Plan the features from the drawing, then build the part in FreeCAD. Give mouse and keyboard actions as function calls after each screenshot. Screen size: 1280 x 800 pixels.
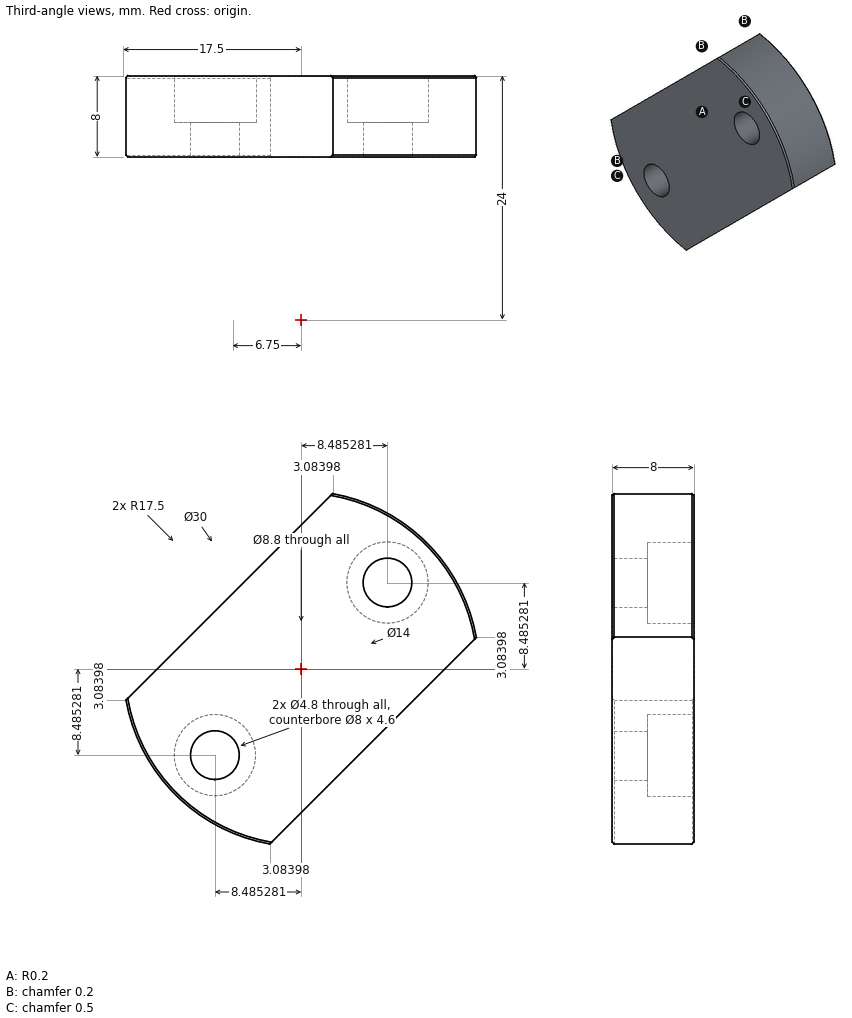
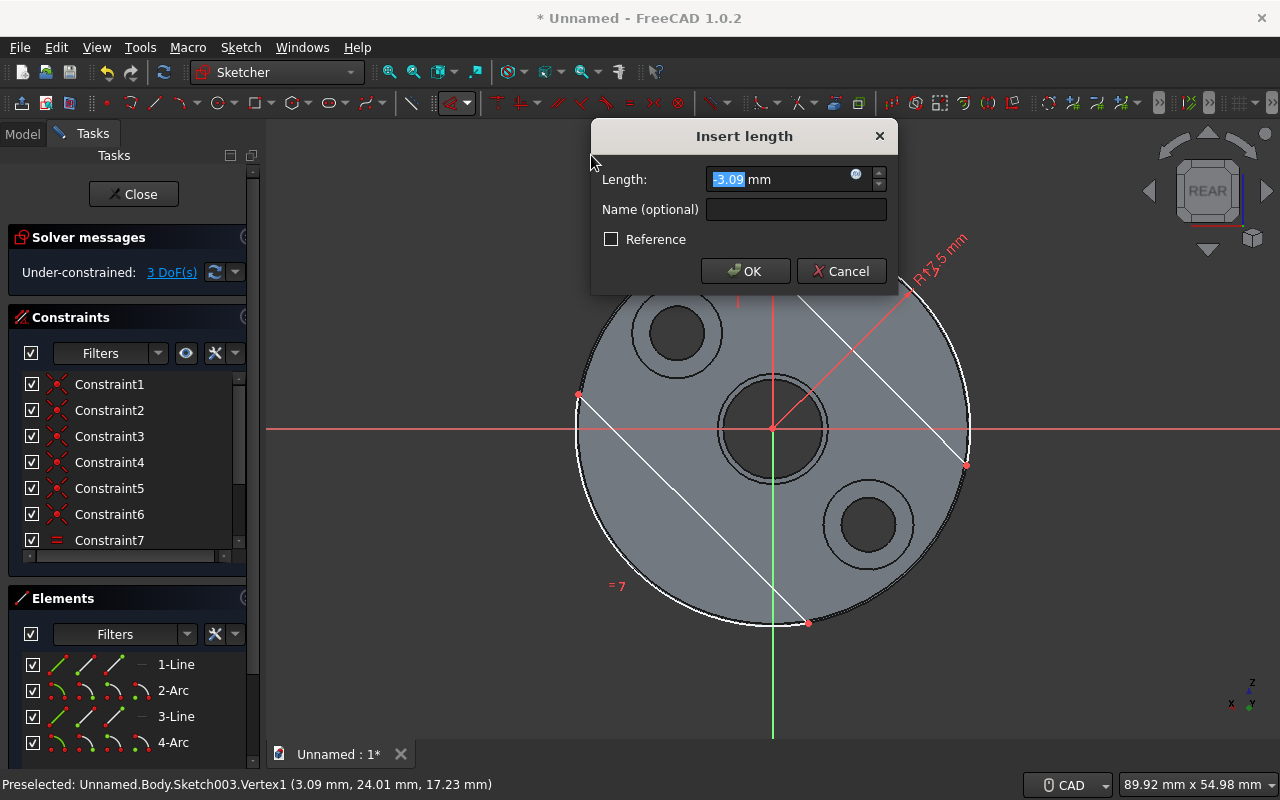
text(-3.08398)
key(Return)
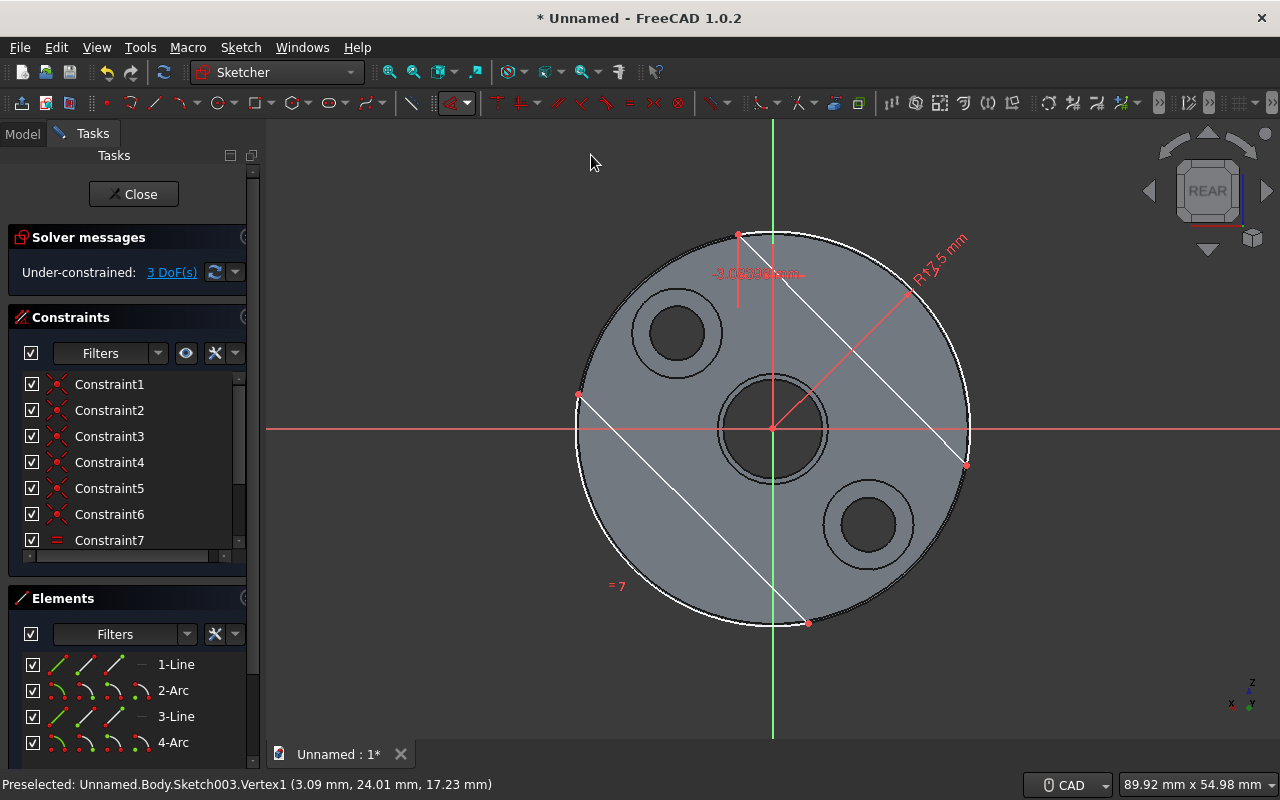
click(967, 465)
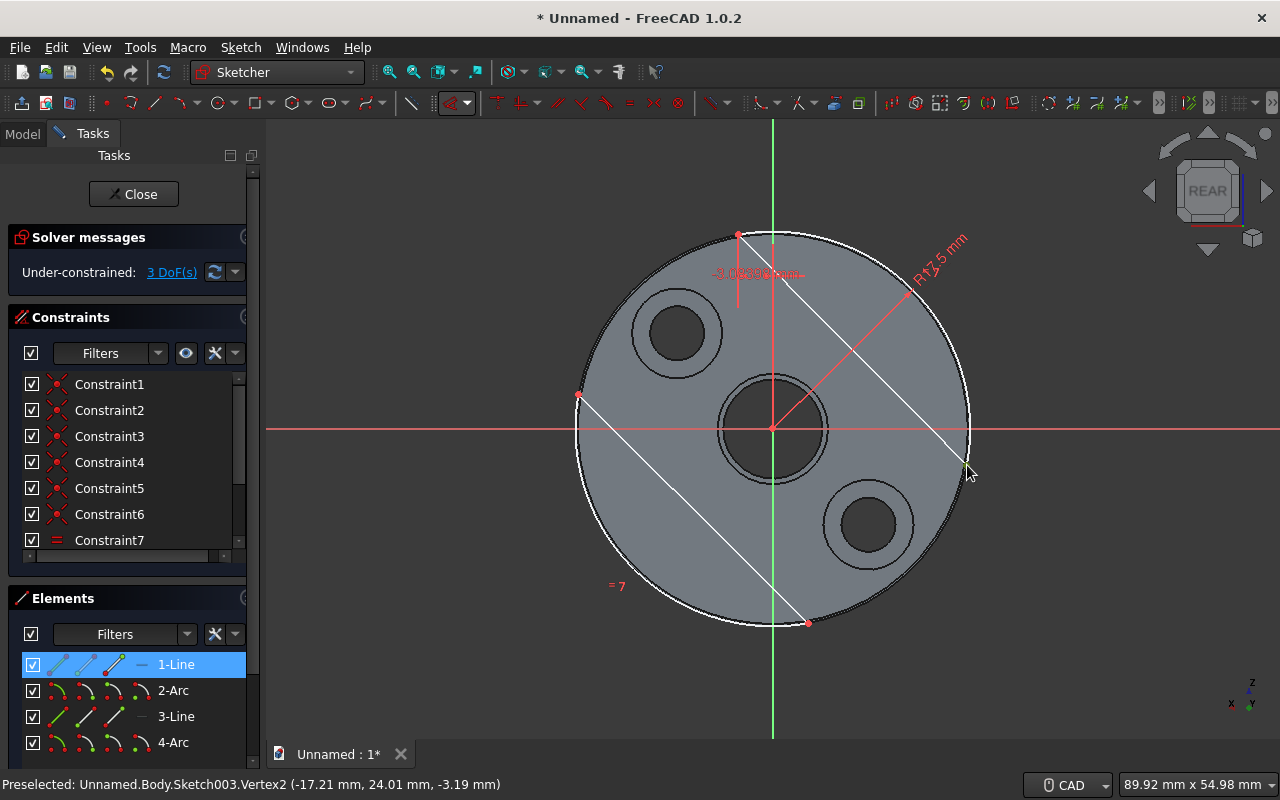
click(470, 104)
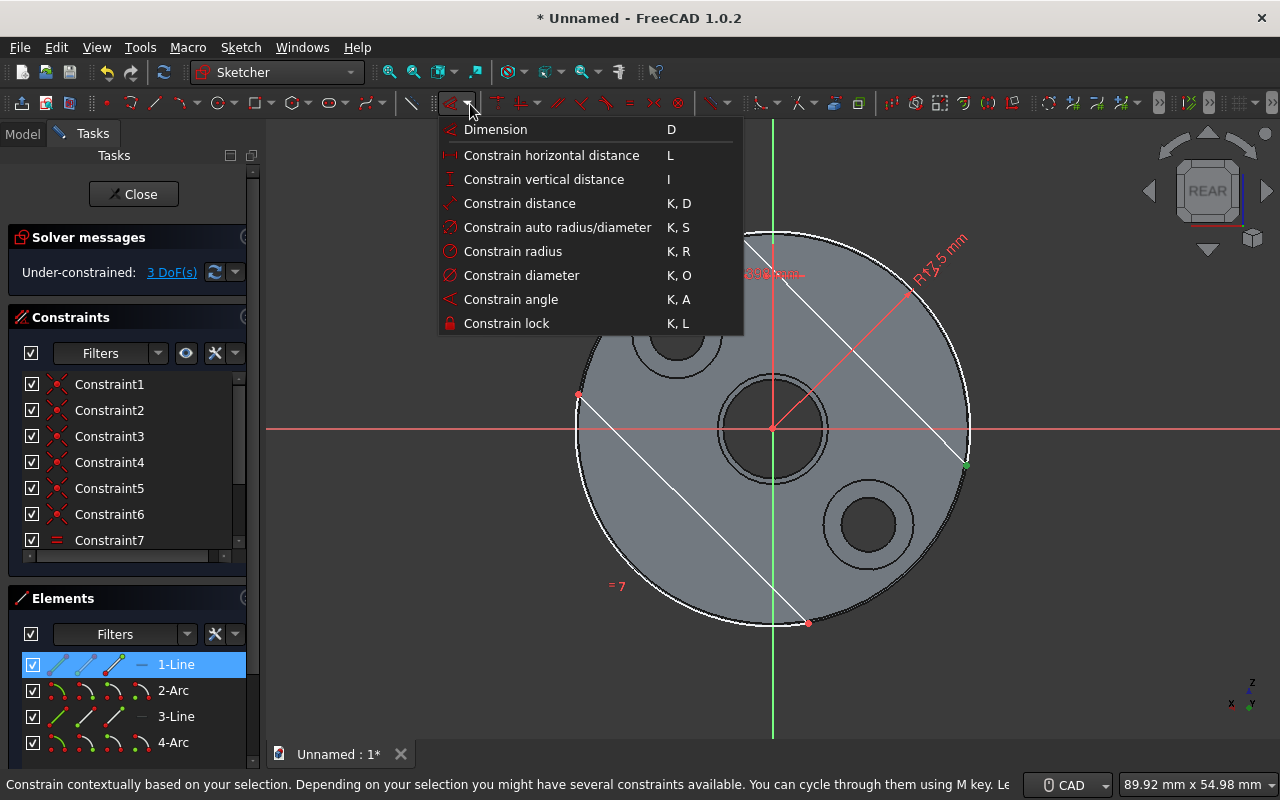
click(591, 179)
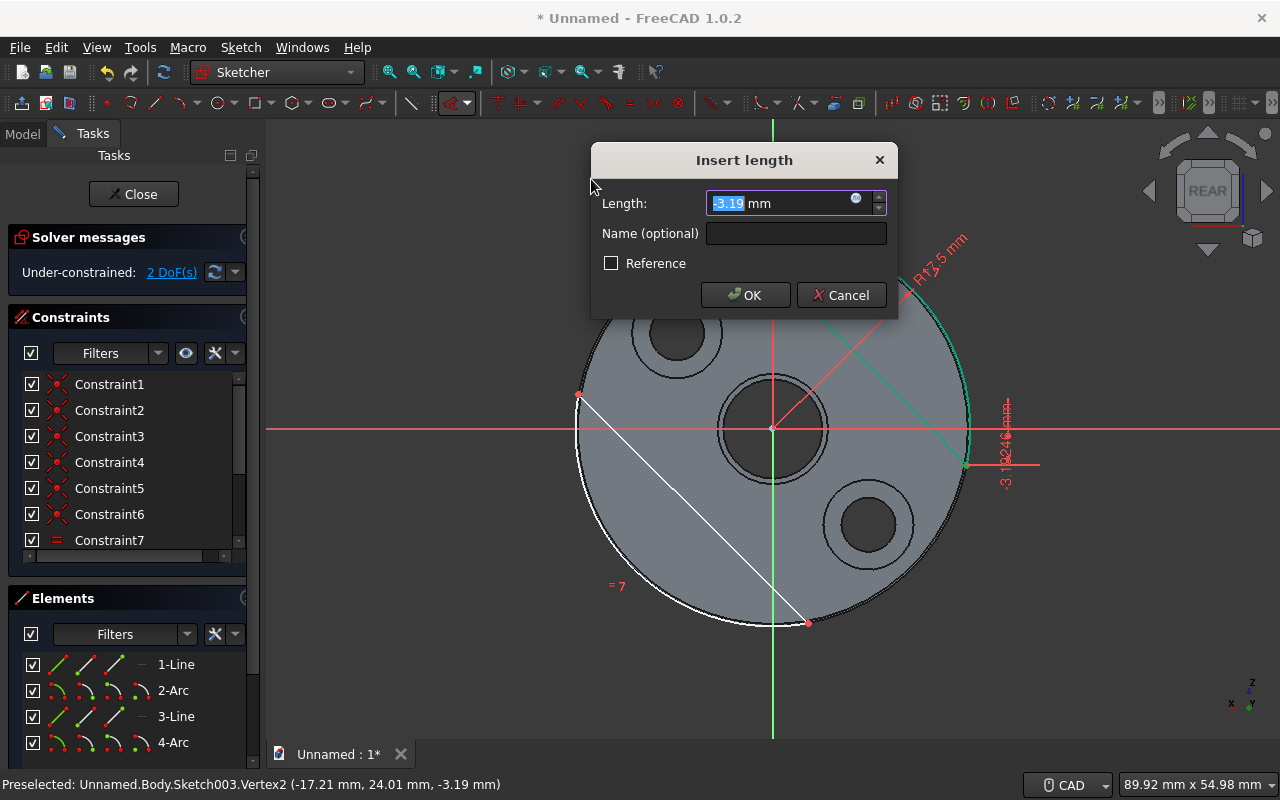
text(-3.08398)
key(Return)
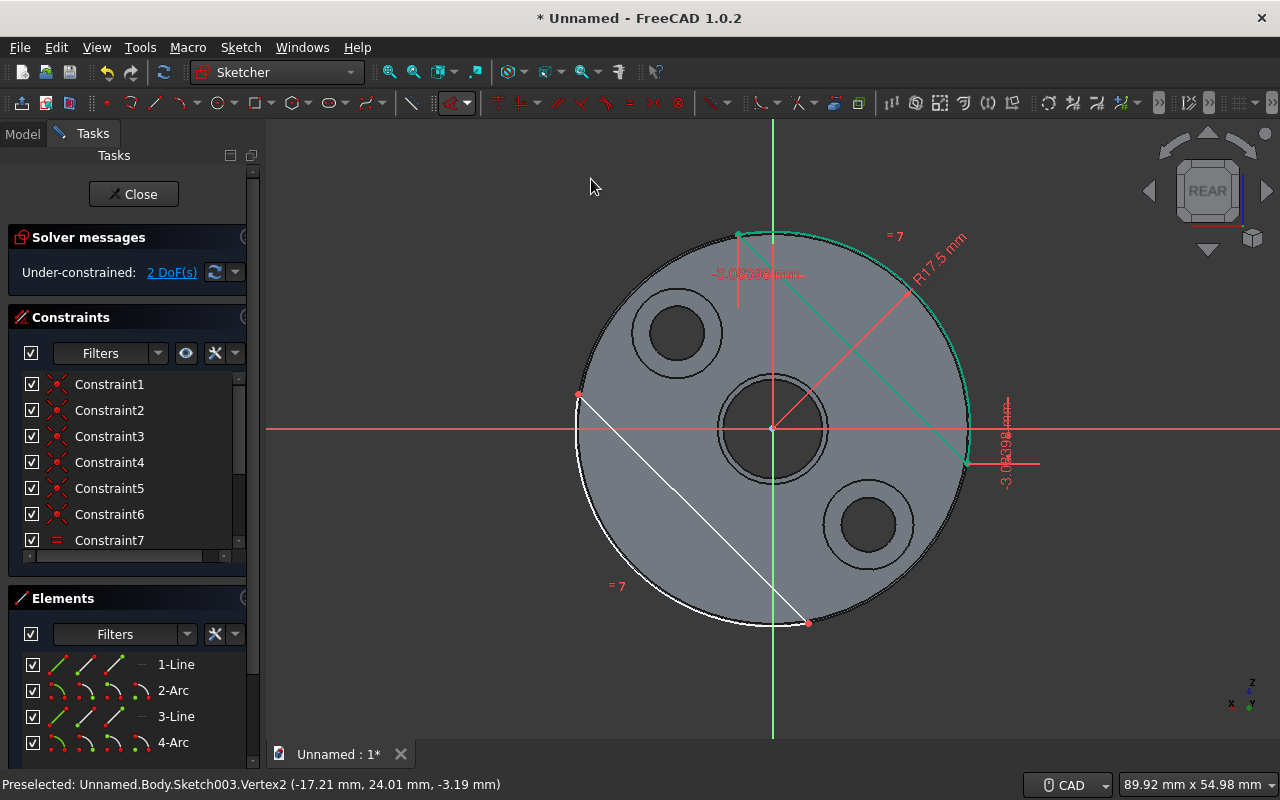
click(808, 623)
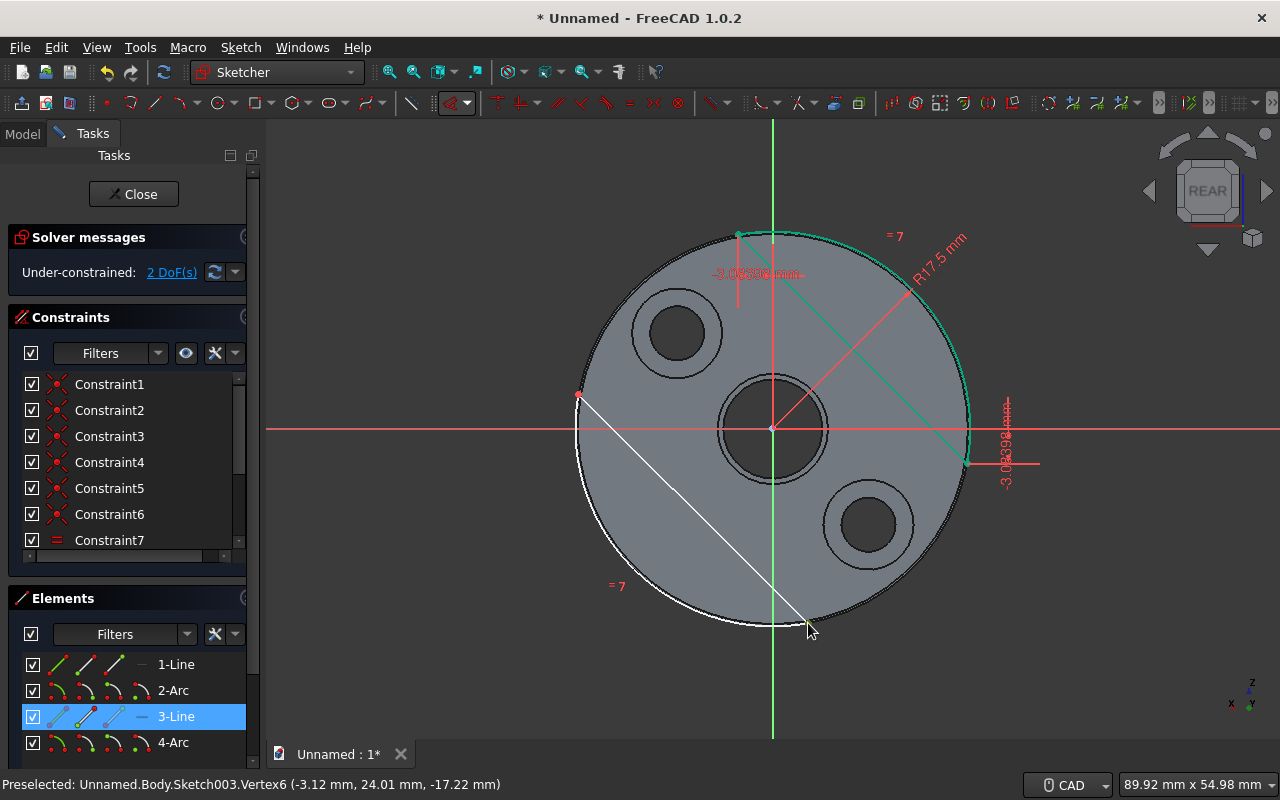
key(l)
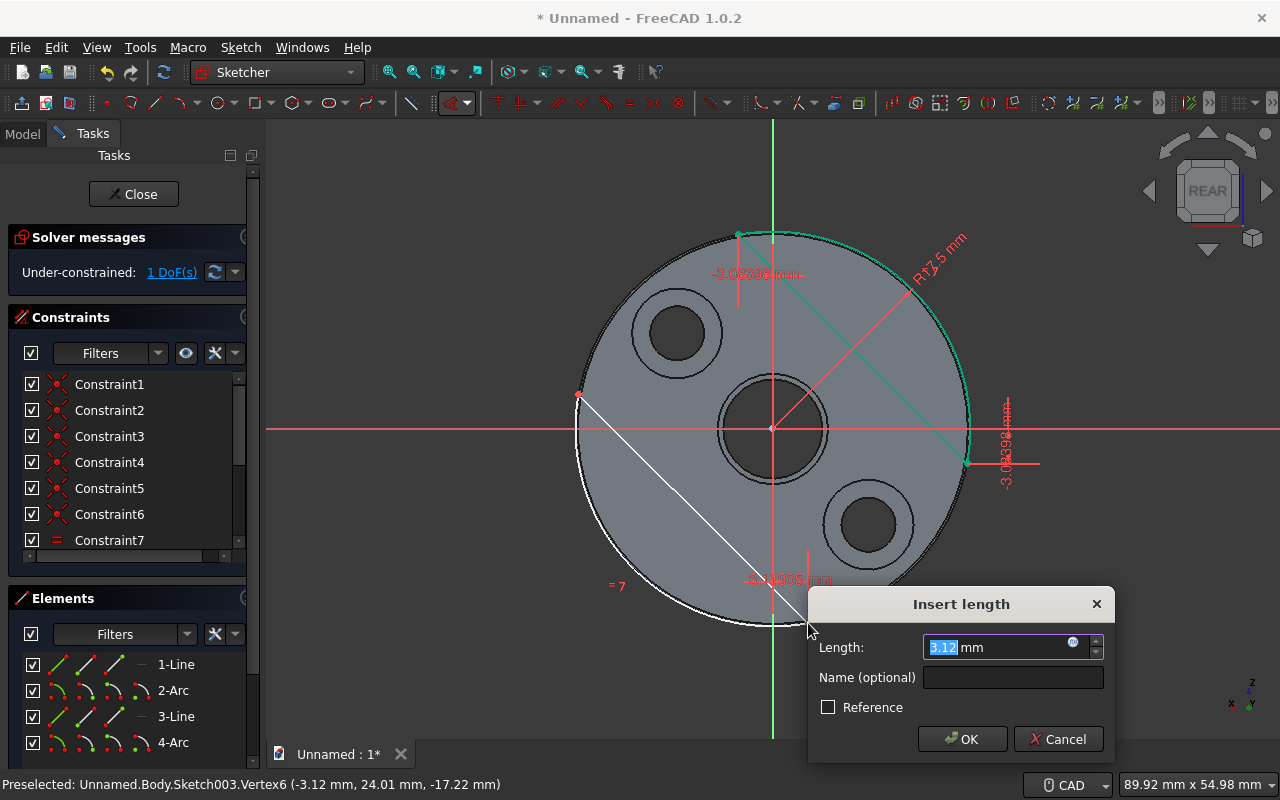
text(3.08398)
key(Return)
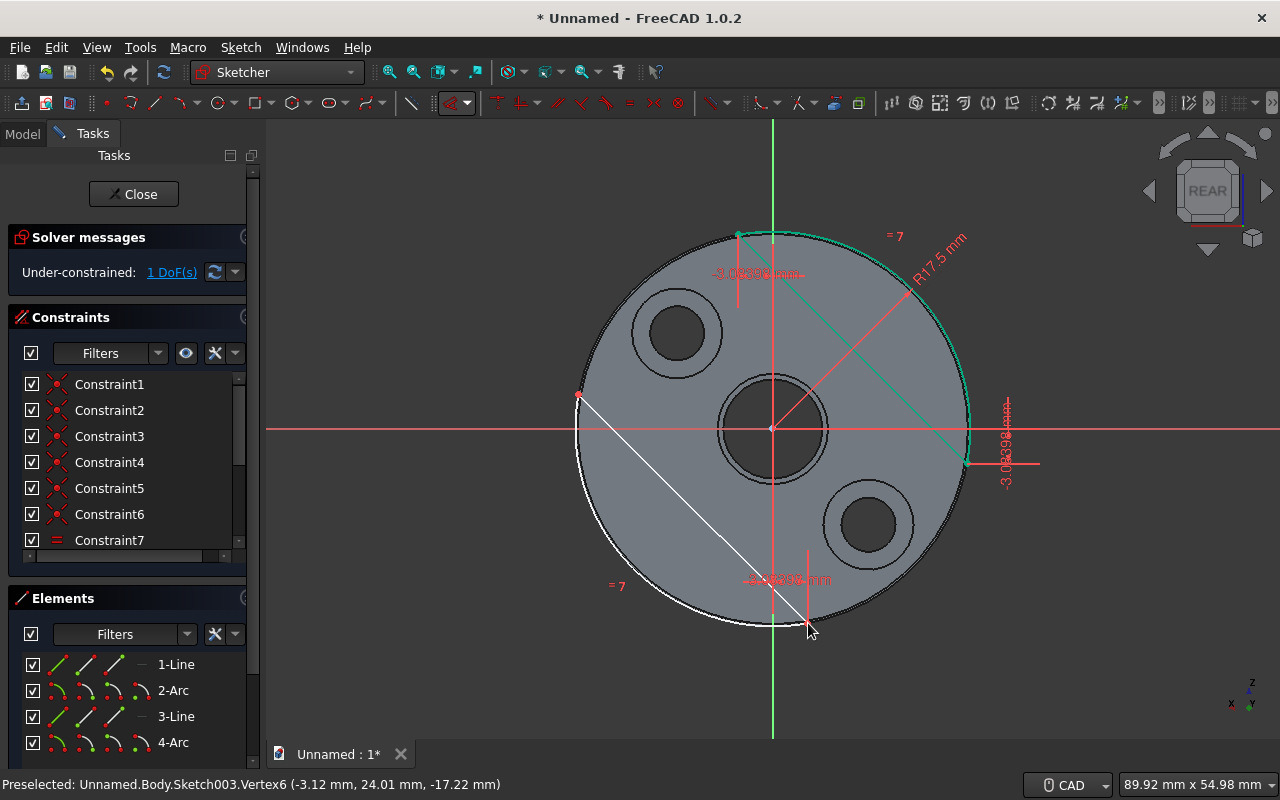
click(578, 395)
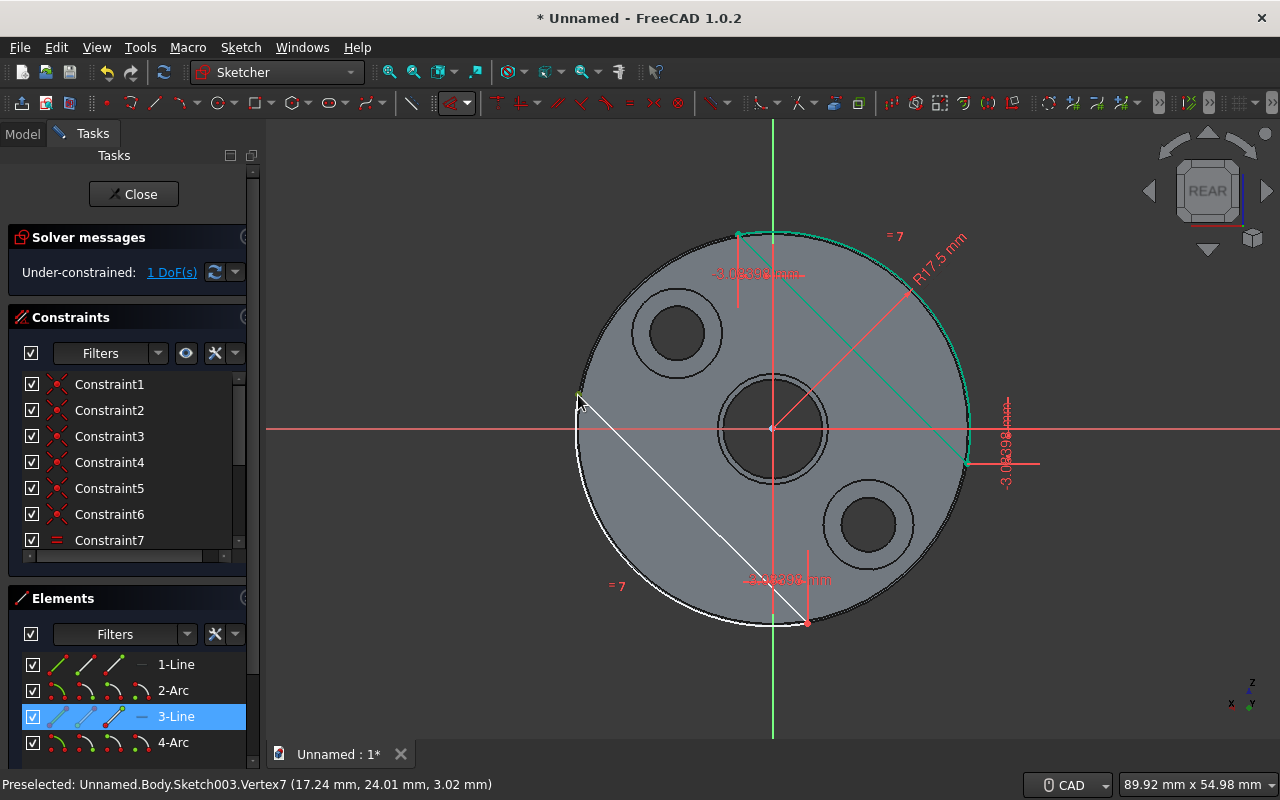
key(i)